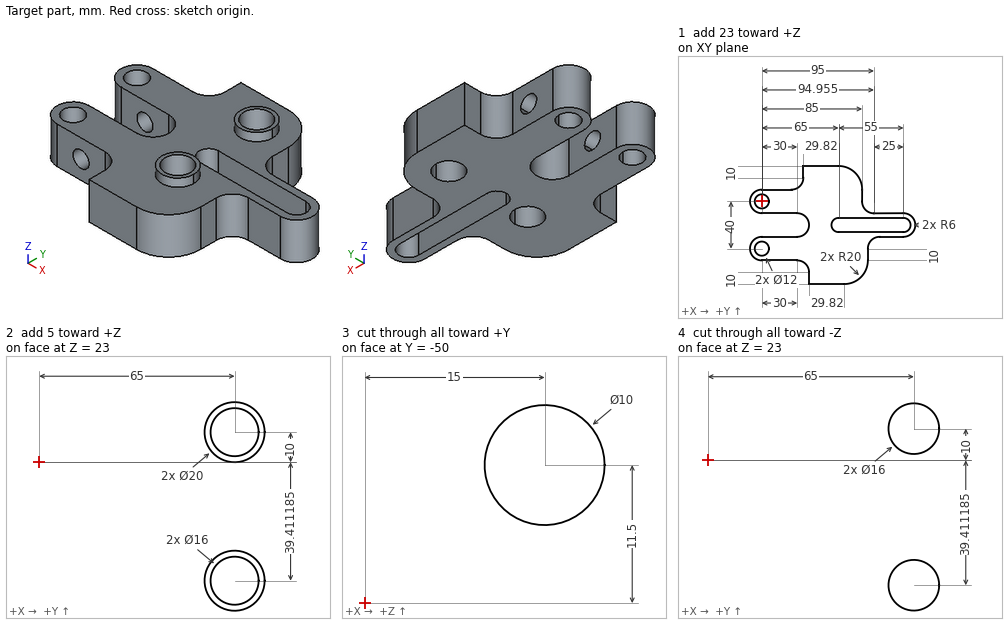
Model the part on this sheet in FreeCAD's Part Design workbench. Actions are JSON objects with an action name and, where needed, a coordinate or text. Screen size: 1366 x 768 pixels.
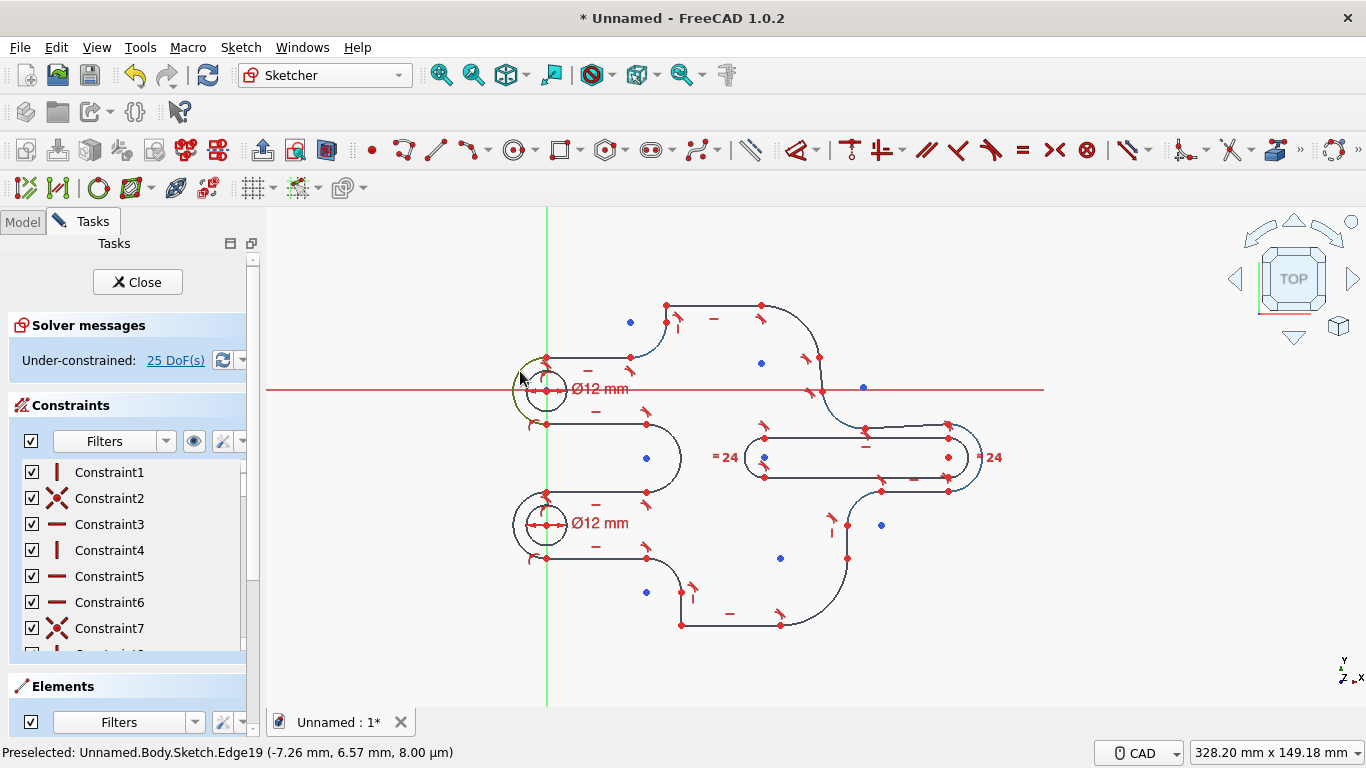
{"action": "left_click", "coordinate": [674, 478]}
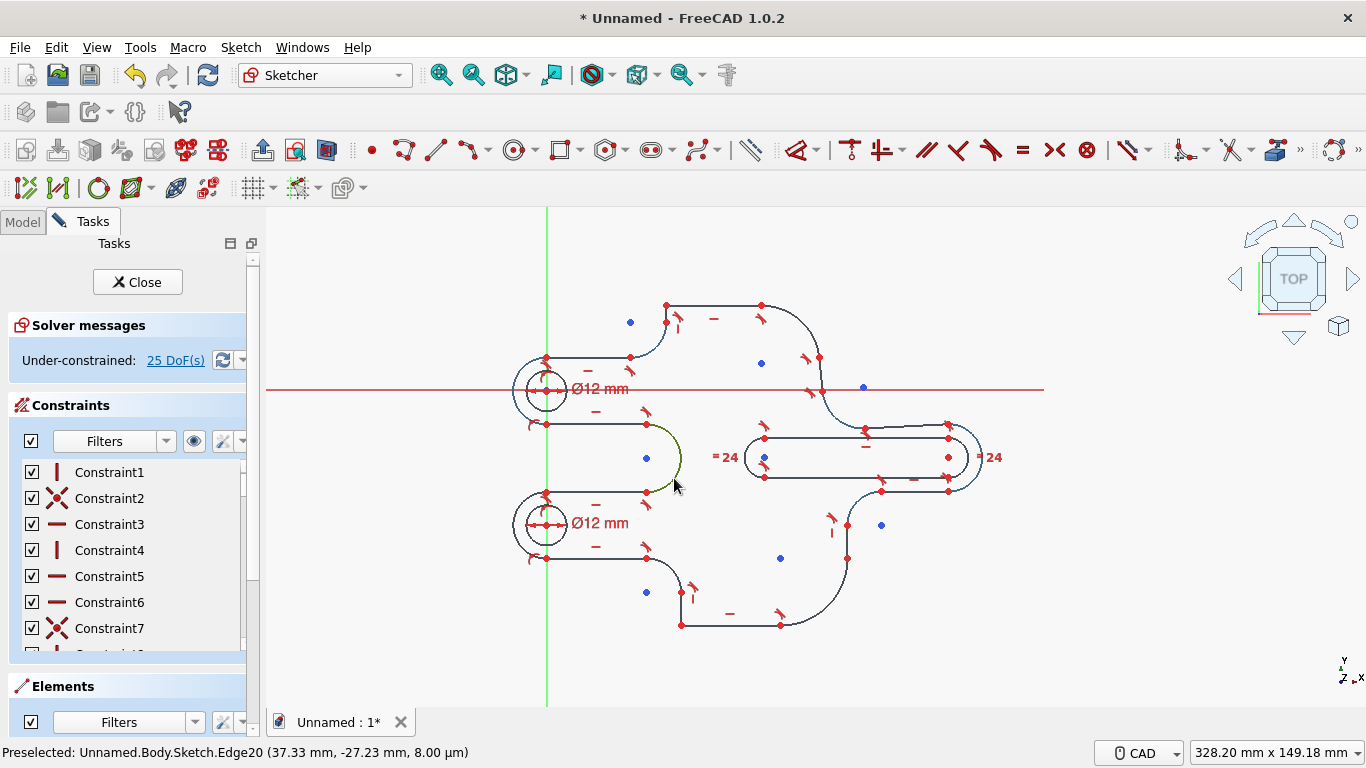
{"action": "left_click", "coordinate": [520, 506]}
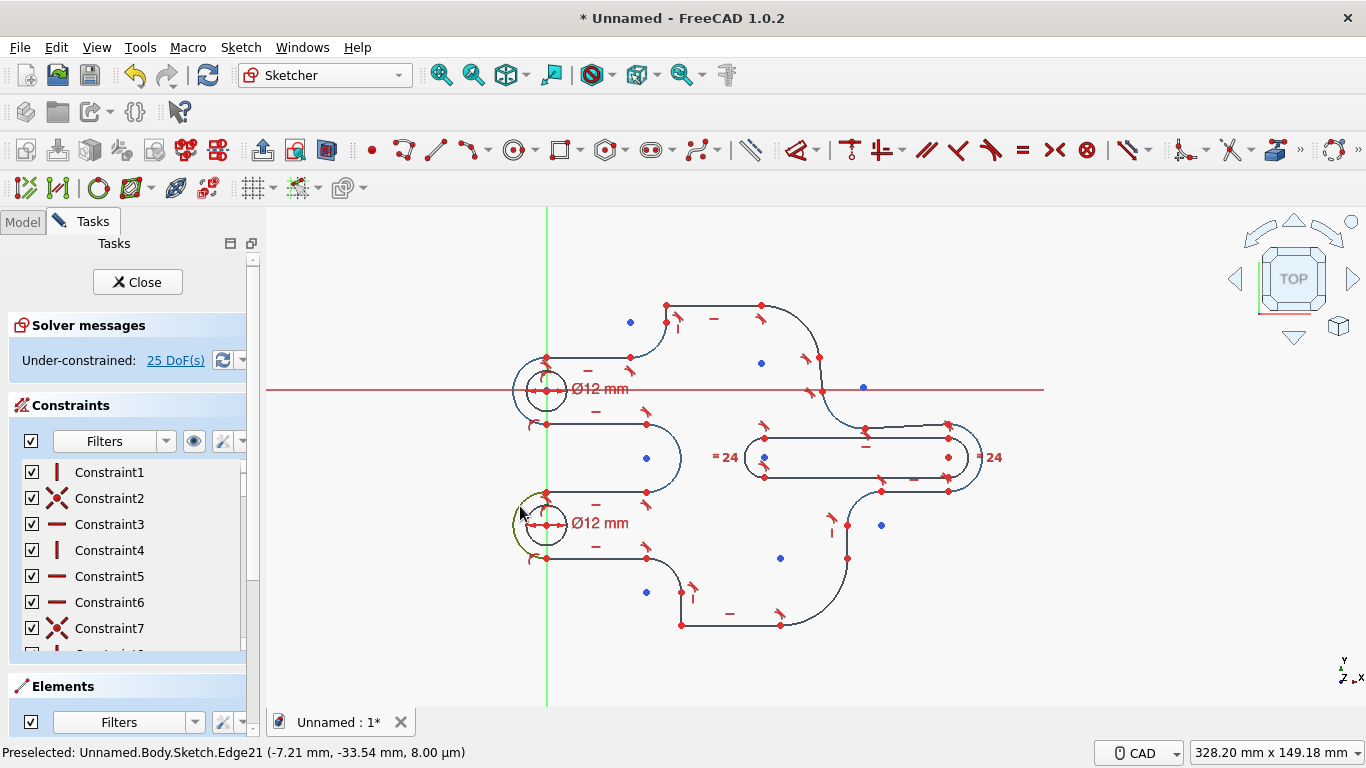
{"action": "left_click", "coordinate": [677, 577]}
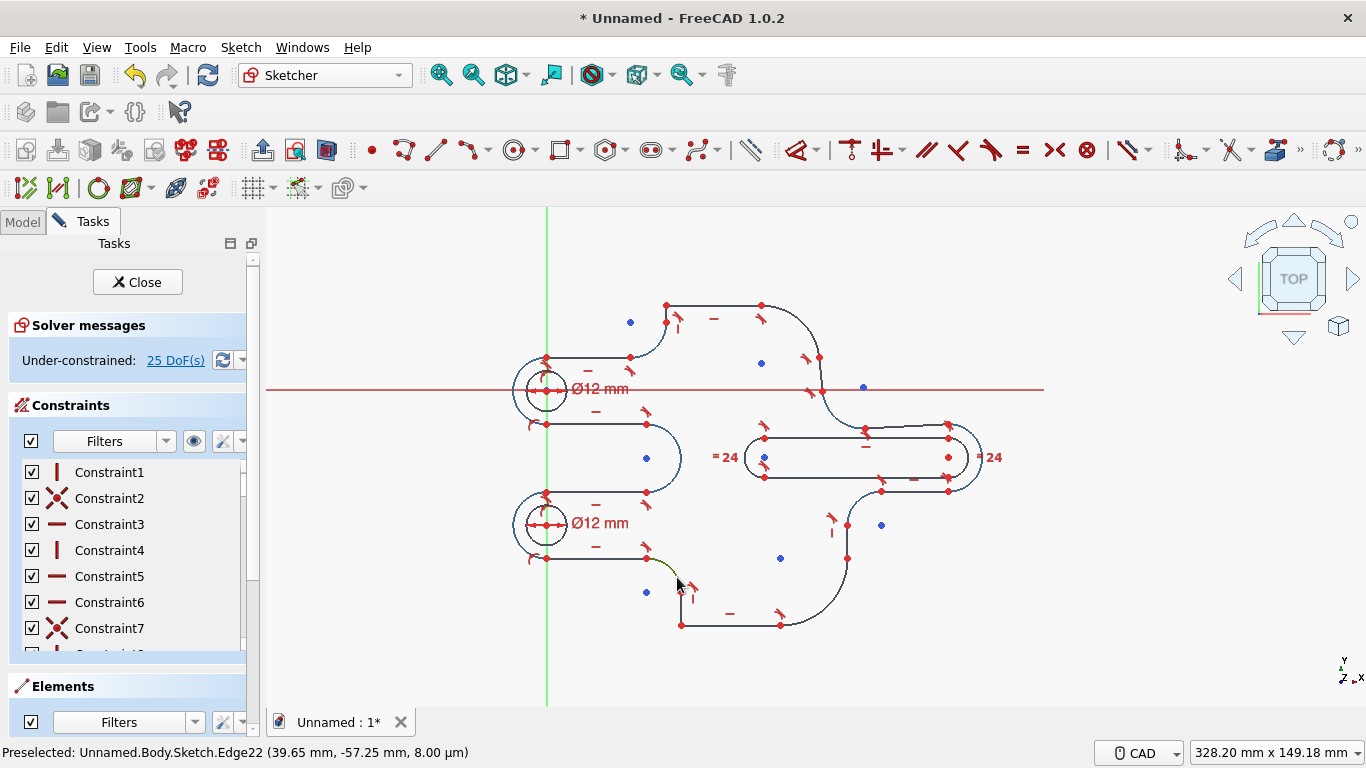
{"action": "left_click", "coordinate": [1024, 150]}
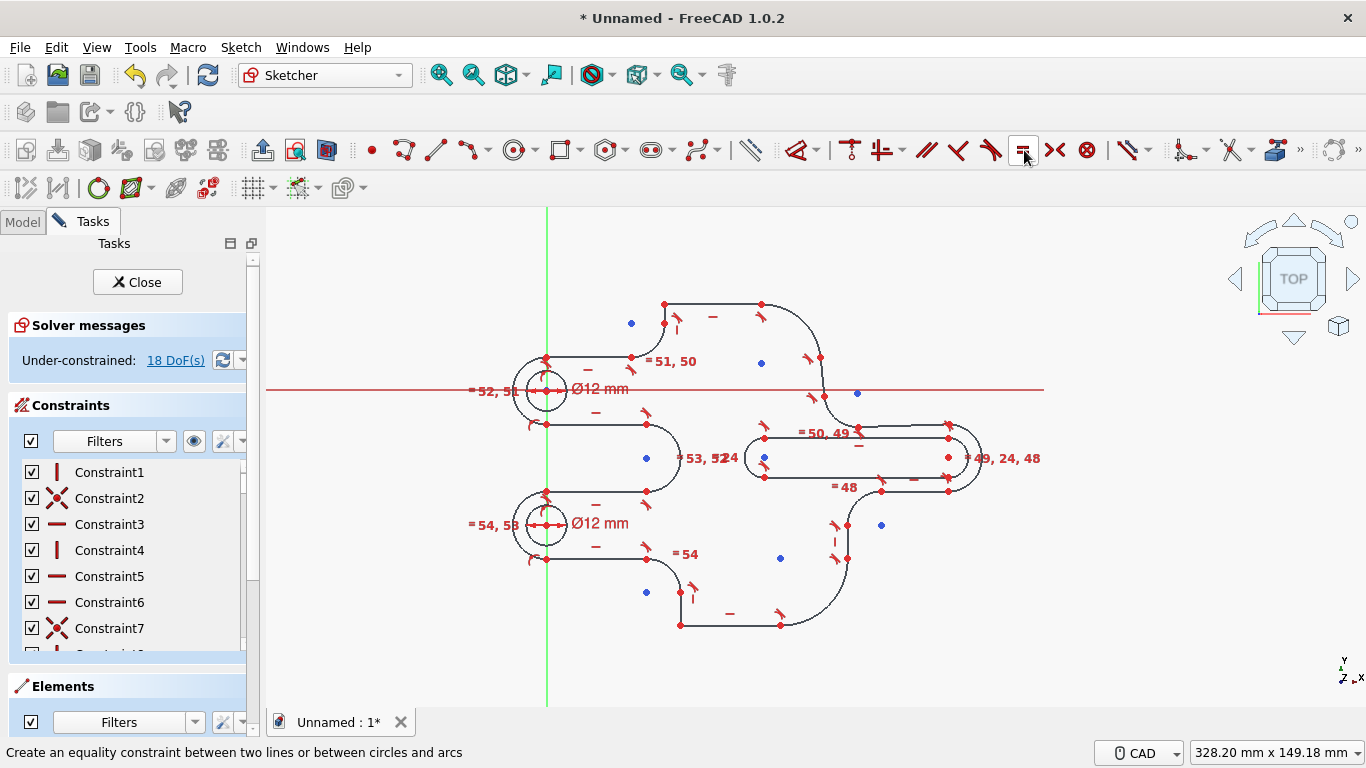
{"action": "left_click", "coordinate": [811, 618]}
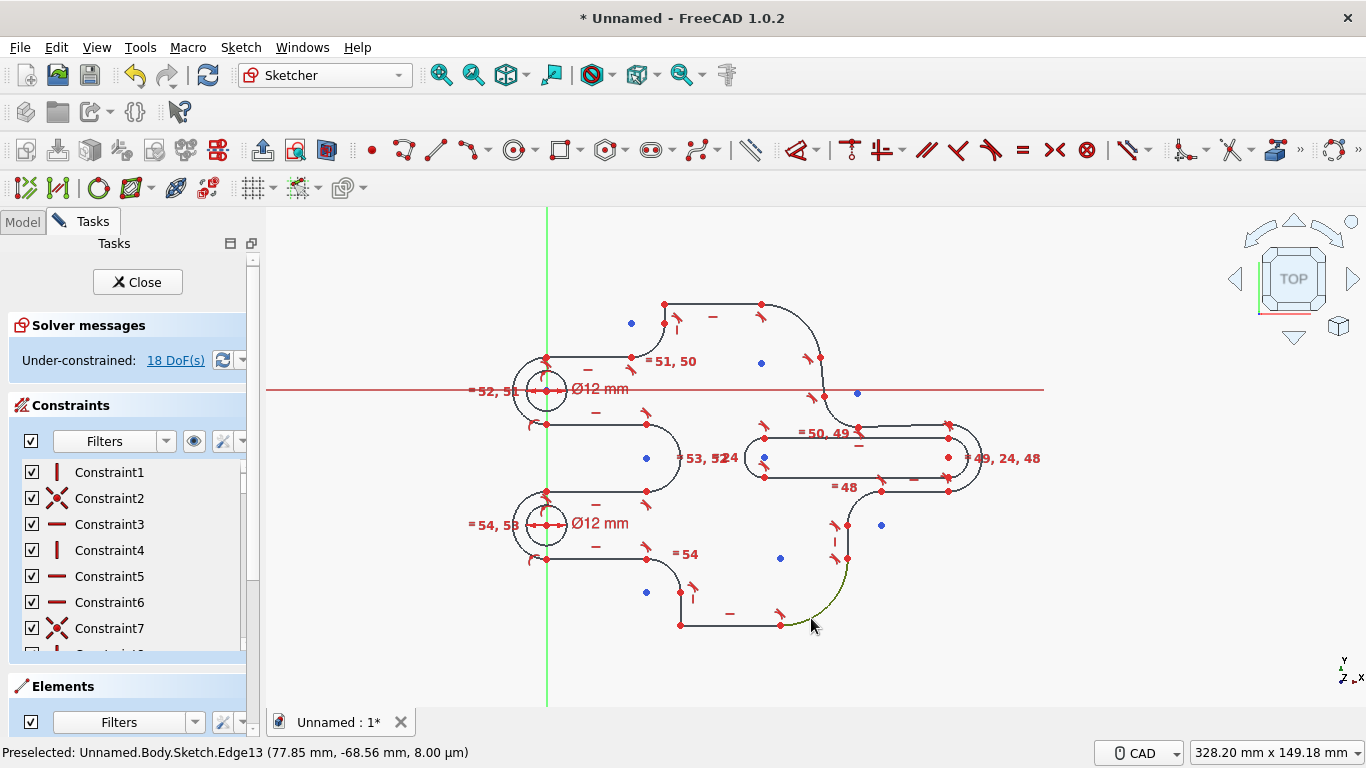
{"action": "left_click", "coordinate": [813, 333]}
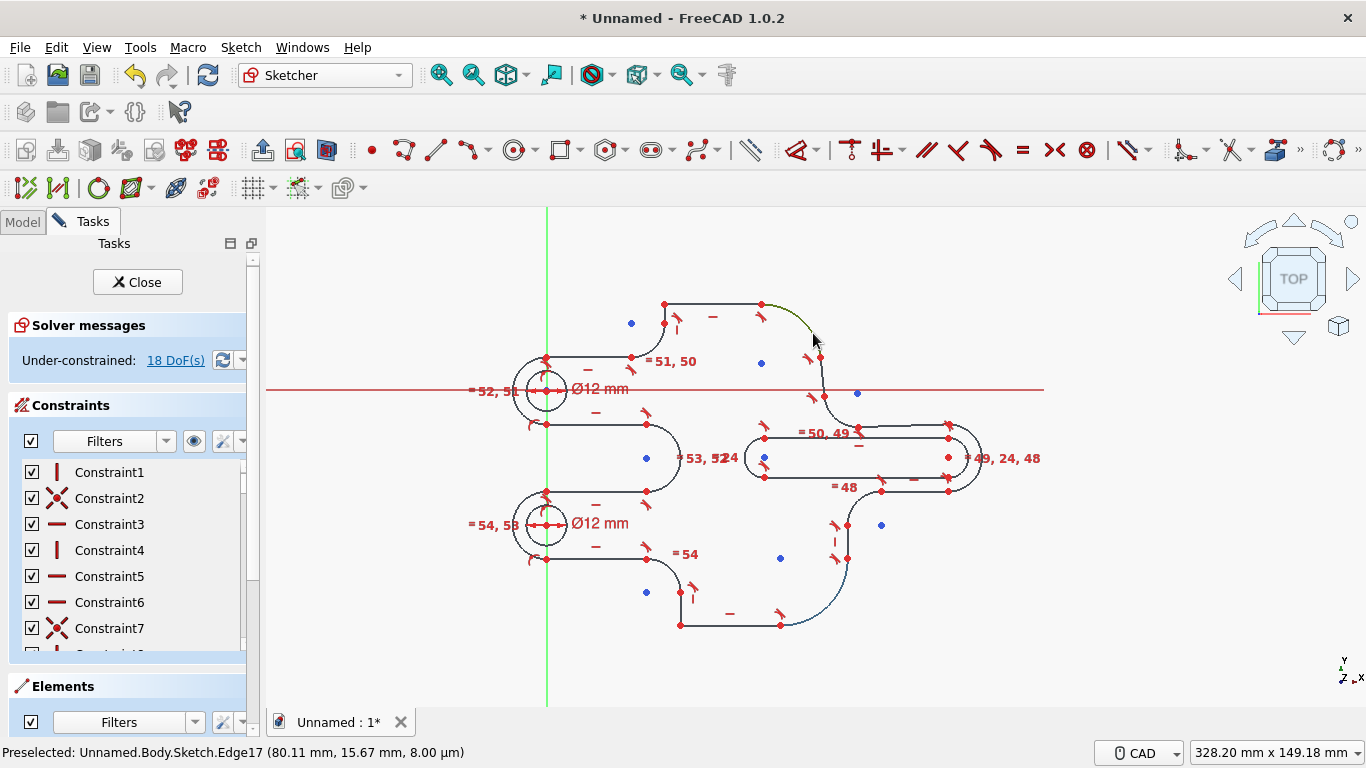
{"action": "left_click", "coordinate": [1024, 150]}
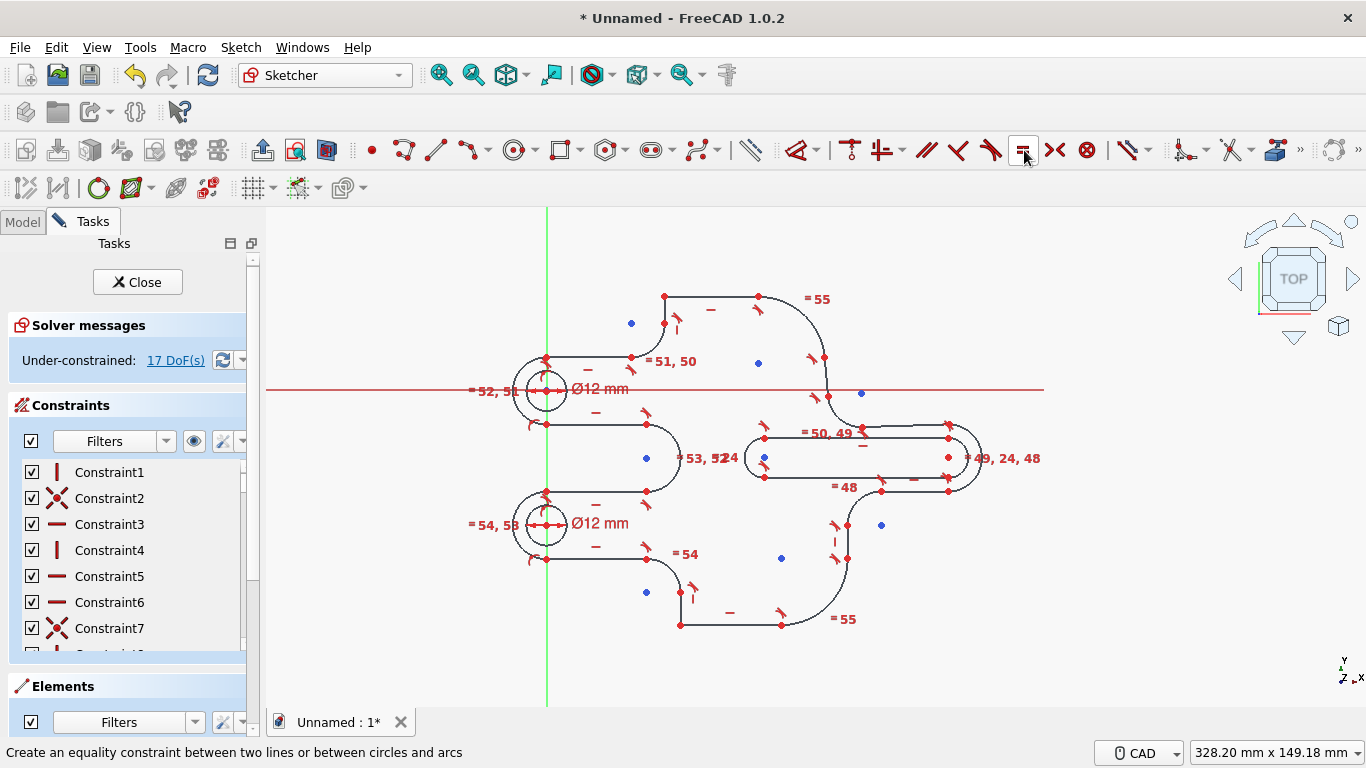
{"action": "left_click", "coordinate": [547, 391]}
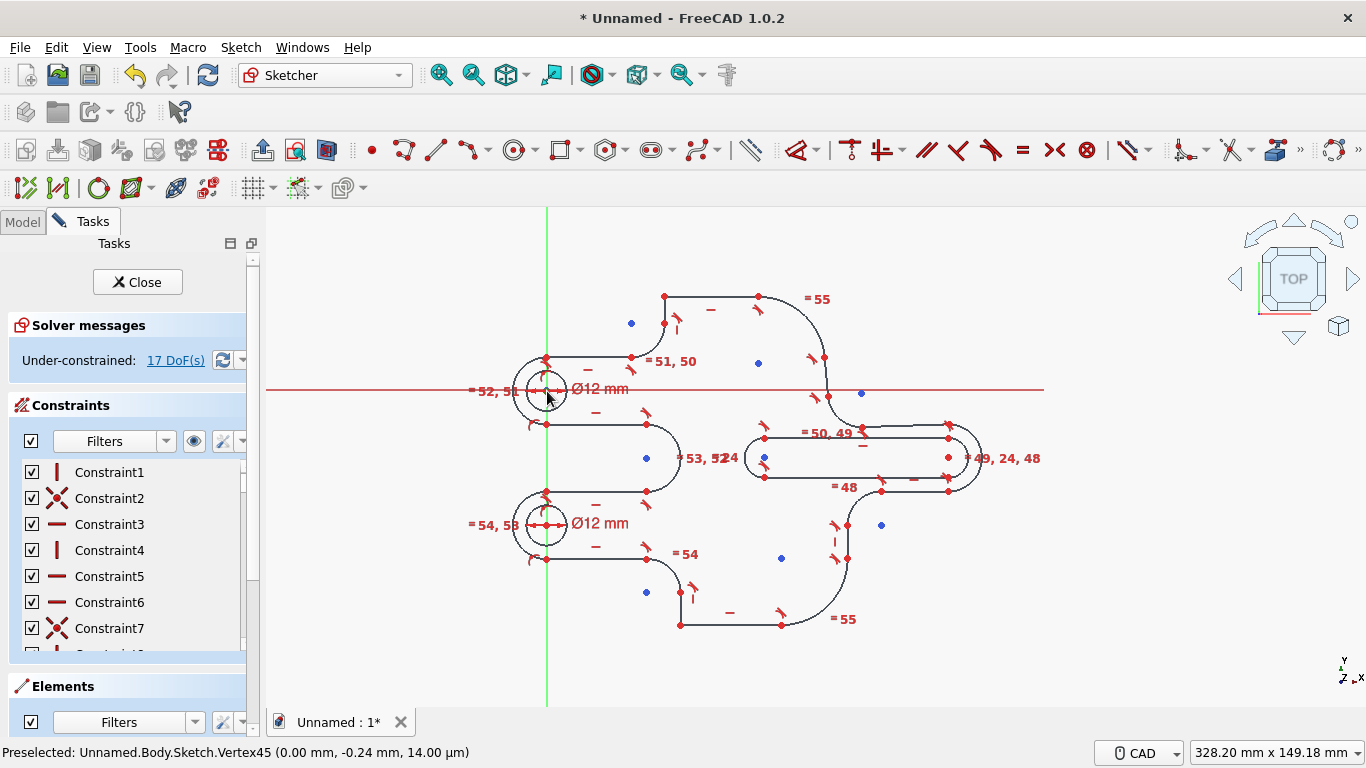
{"action": "left_click", "coordinate": [359, 390]}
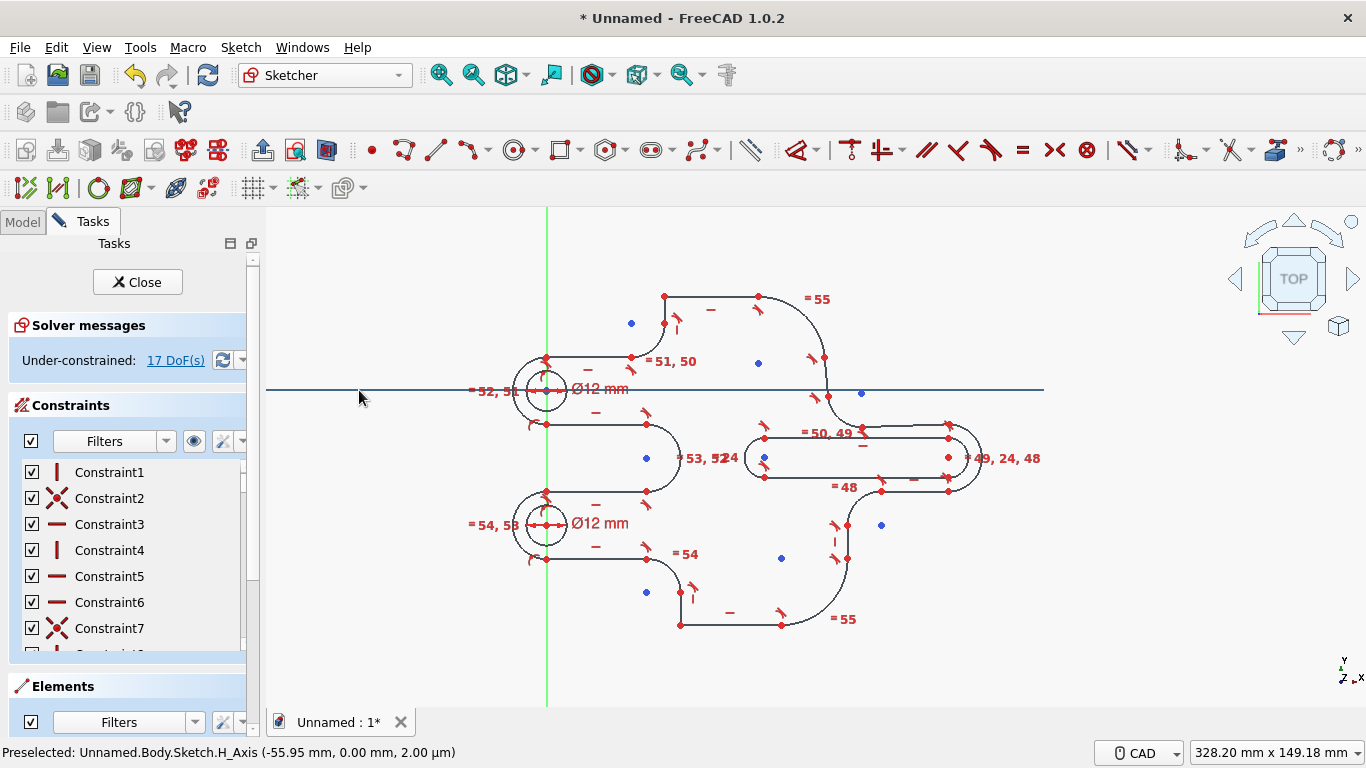
{"action": "left_click", "coordinate": [850, 150]}